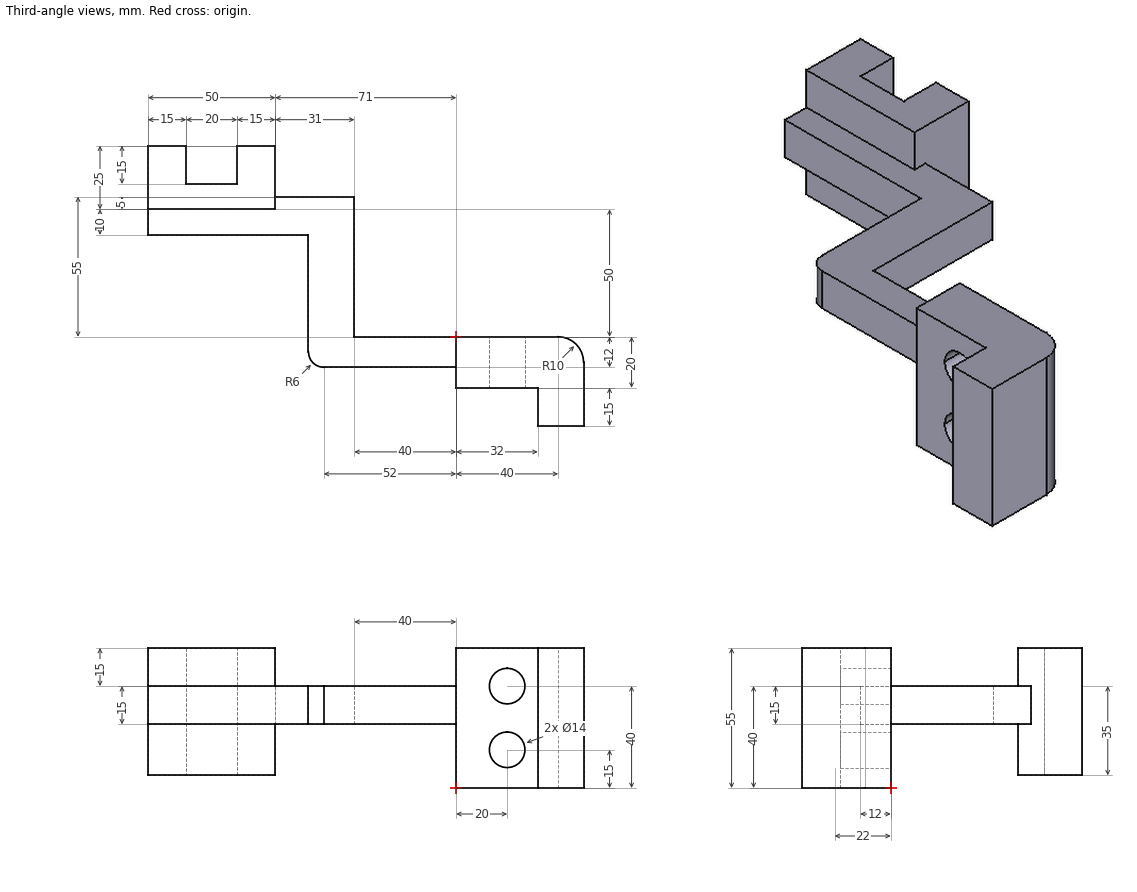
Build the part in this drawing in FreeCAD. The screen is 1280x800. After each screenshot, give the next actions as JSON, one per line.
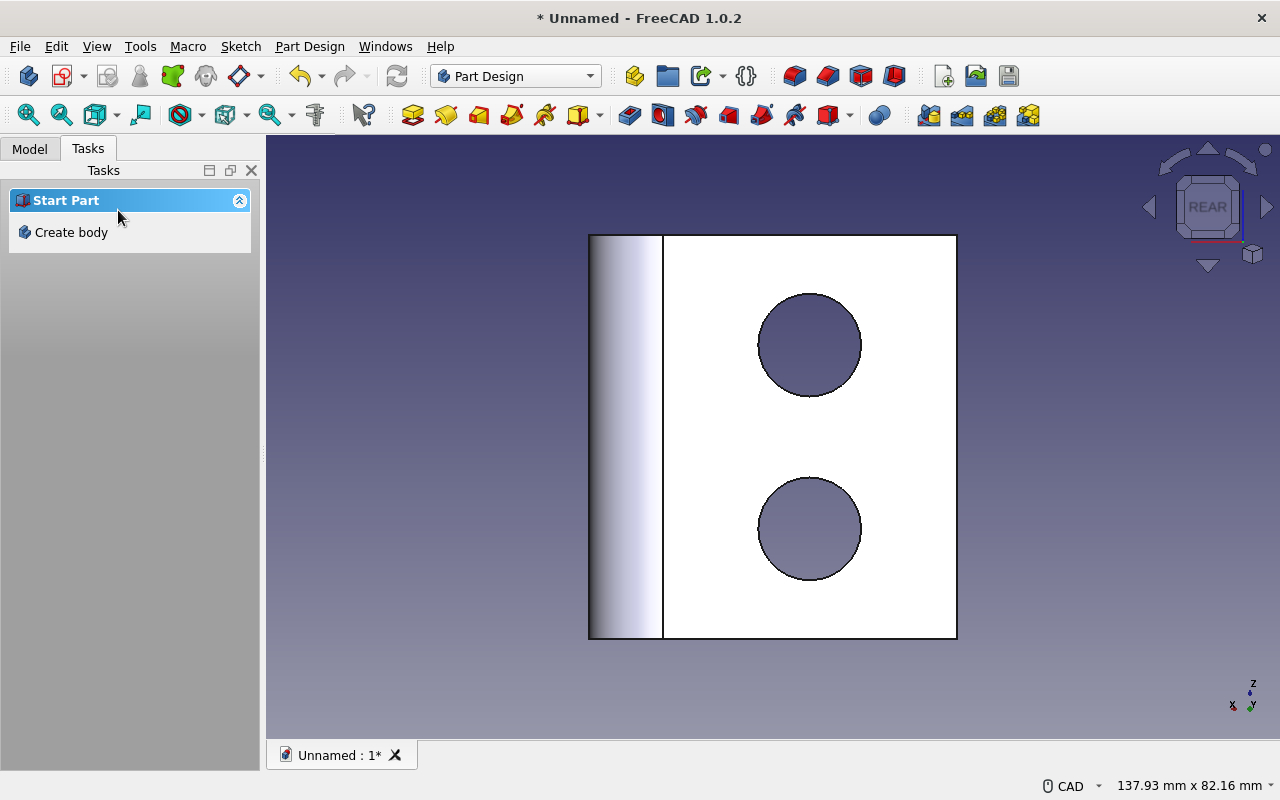
{"action": "left_click", "coordinate": [62, 76]}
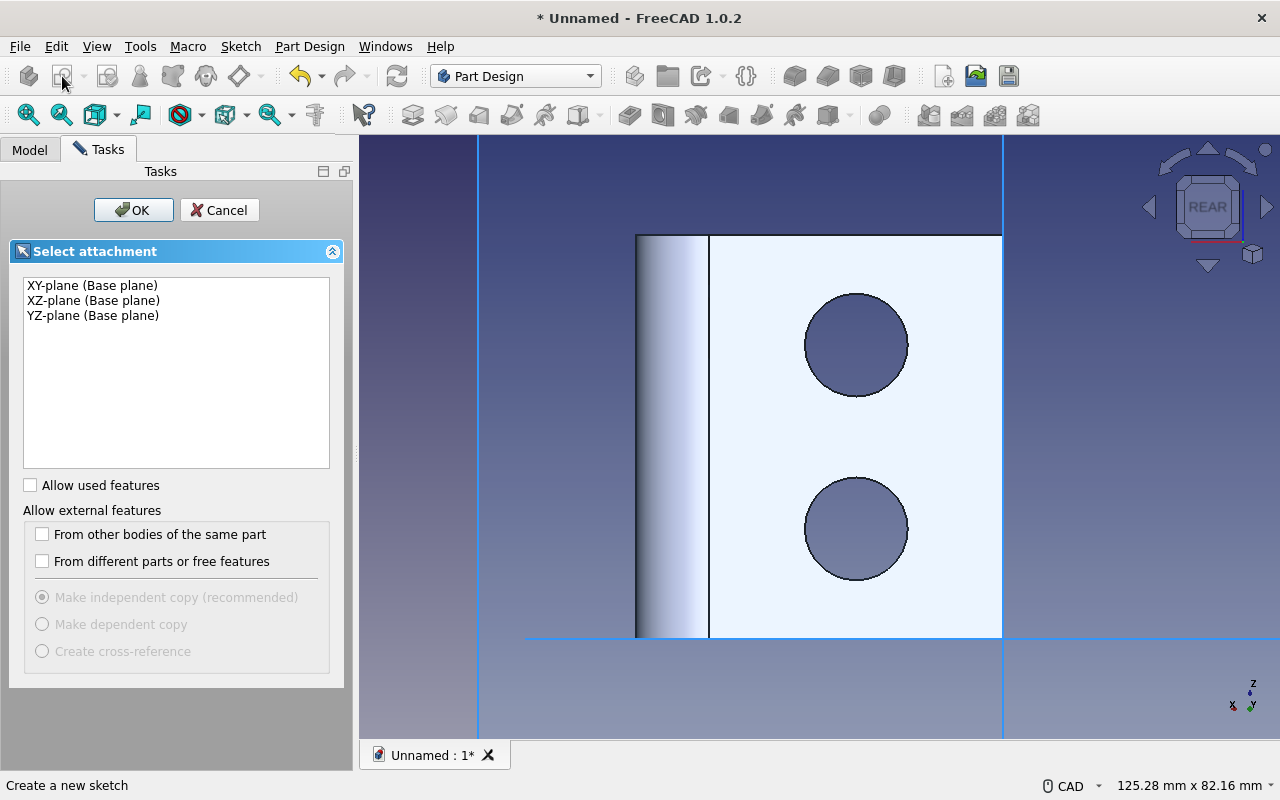
{"action": "left_click", "coordinate": [84, 316]}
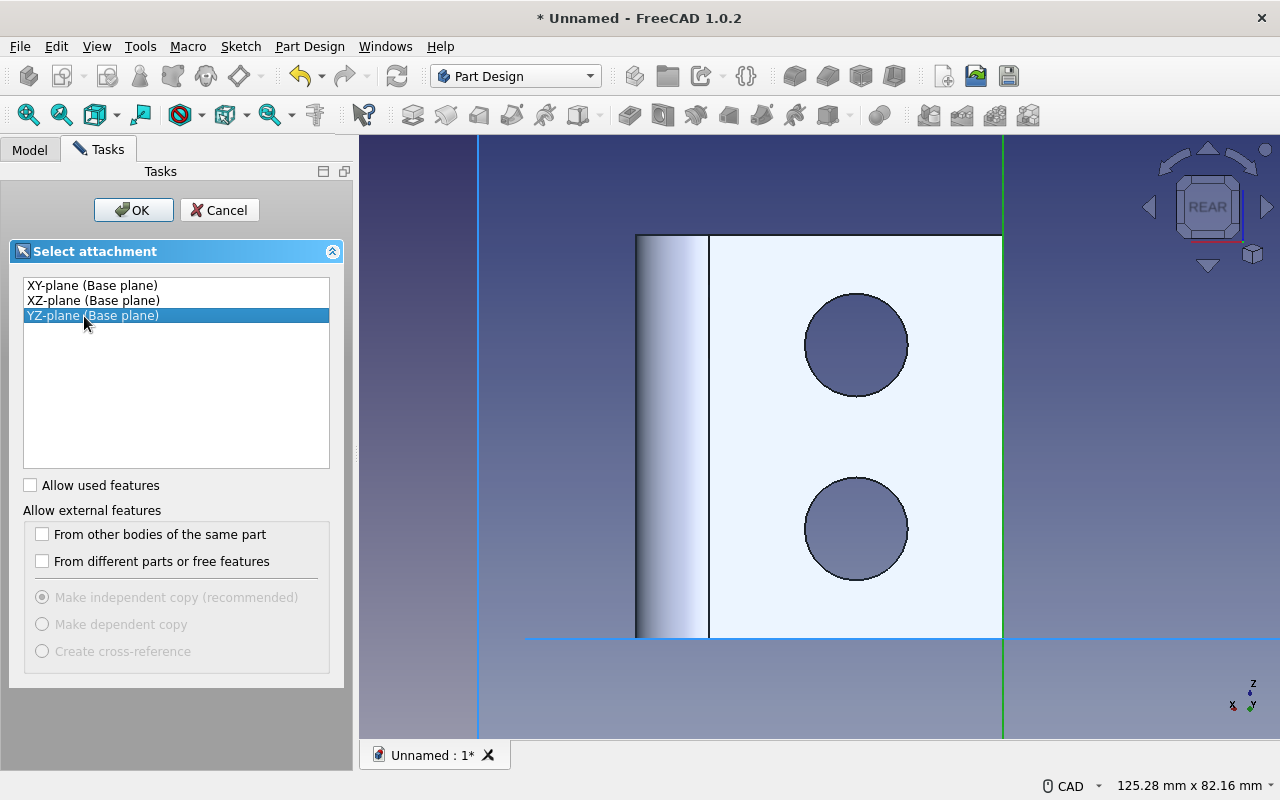
{"action": "left_click", "coordinate": [134, 210]}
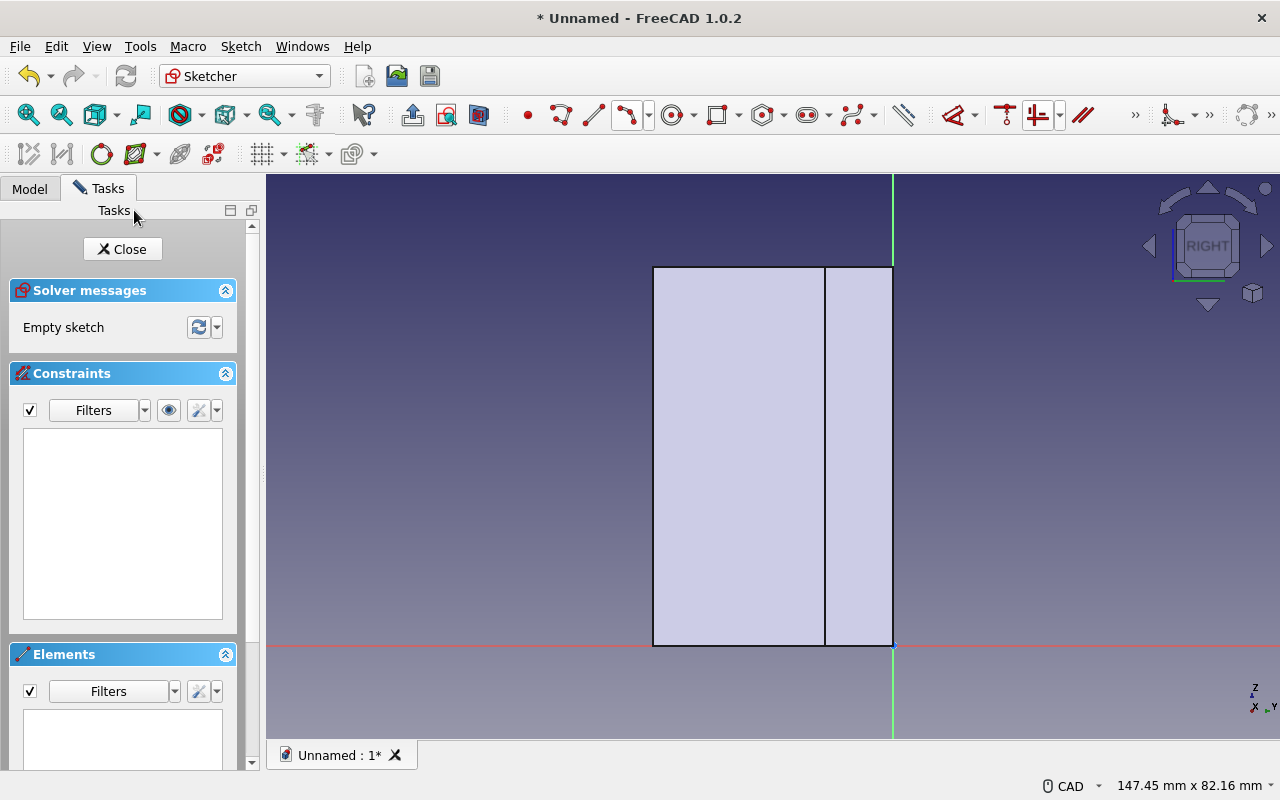
{"action": "left_click", "coordinate": [479, 116]}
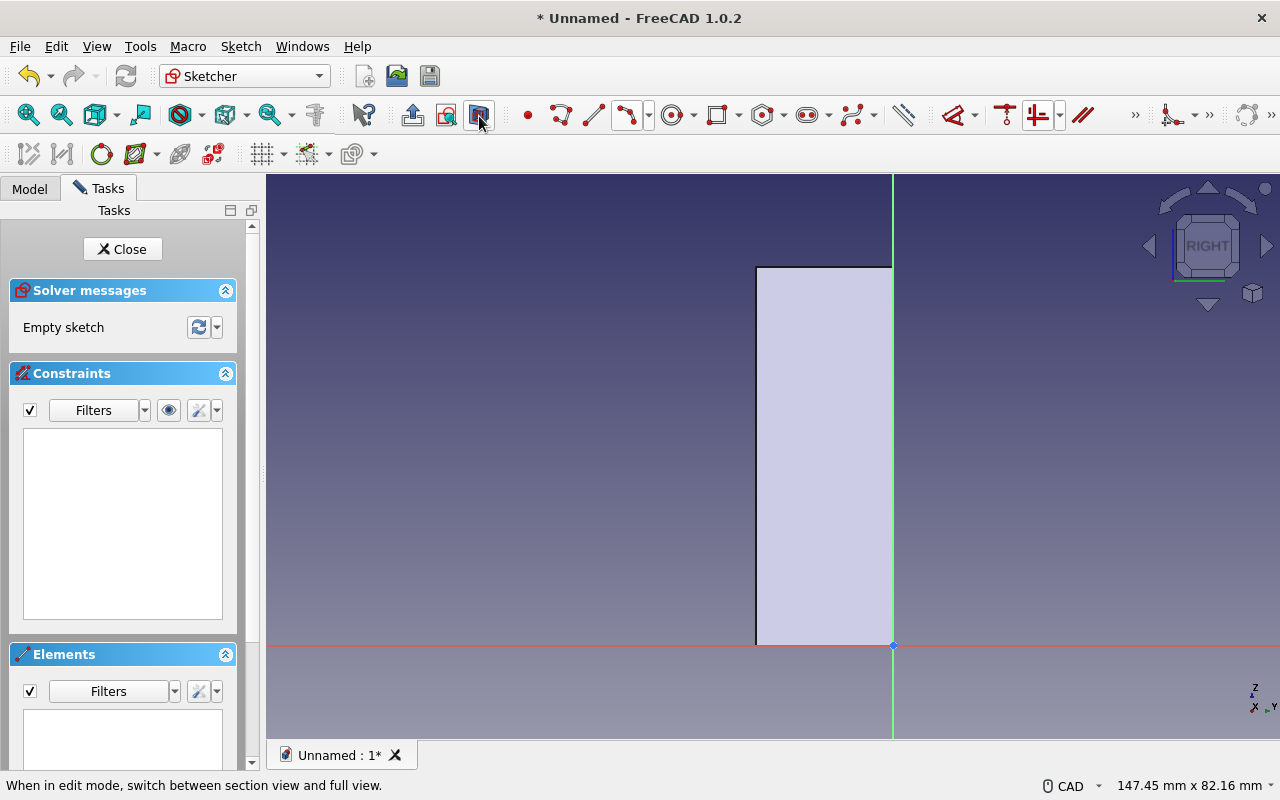
{"action": "scroll", "coordinate": [916, 407], "scroll_direction": "up", "scroll_amount": 6}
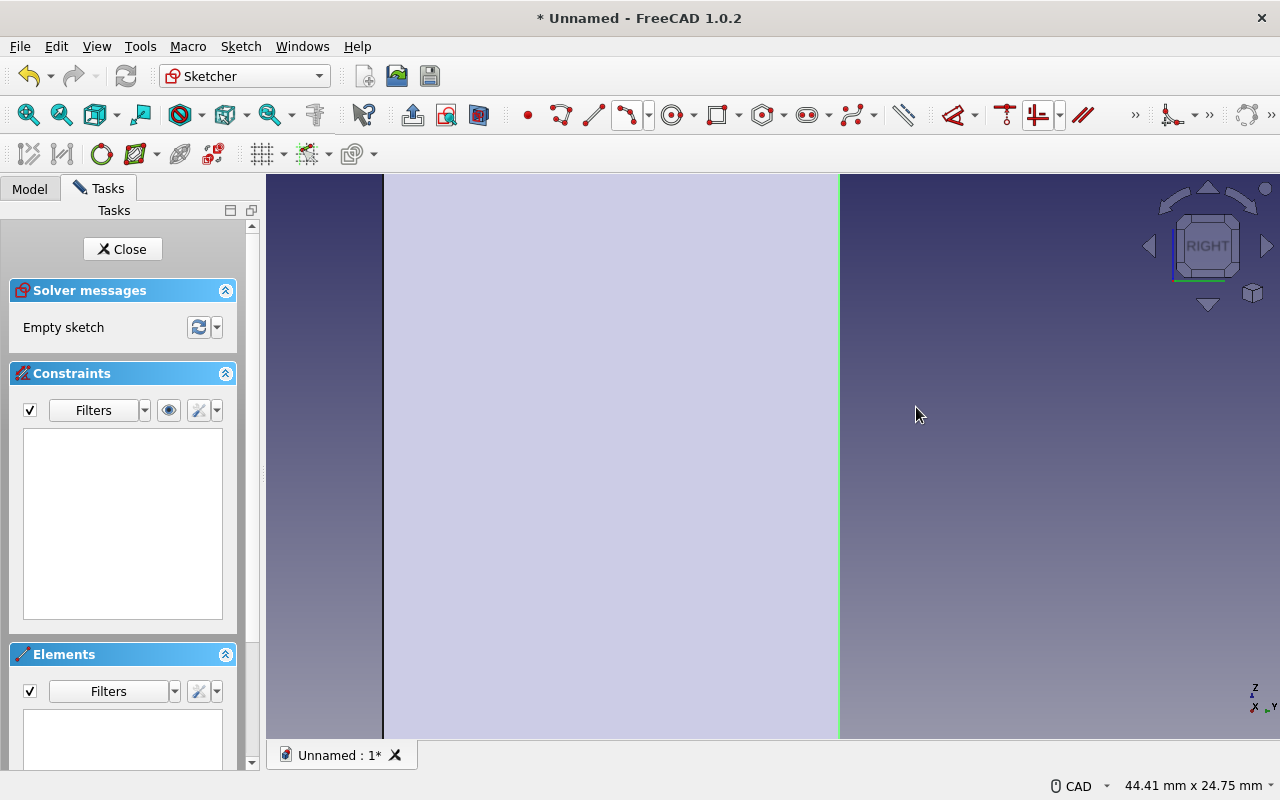
{"action": "left_click", "coordinate": [716, 116]}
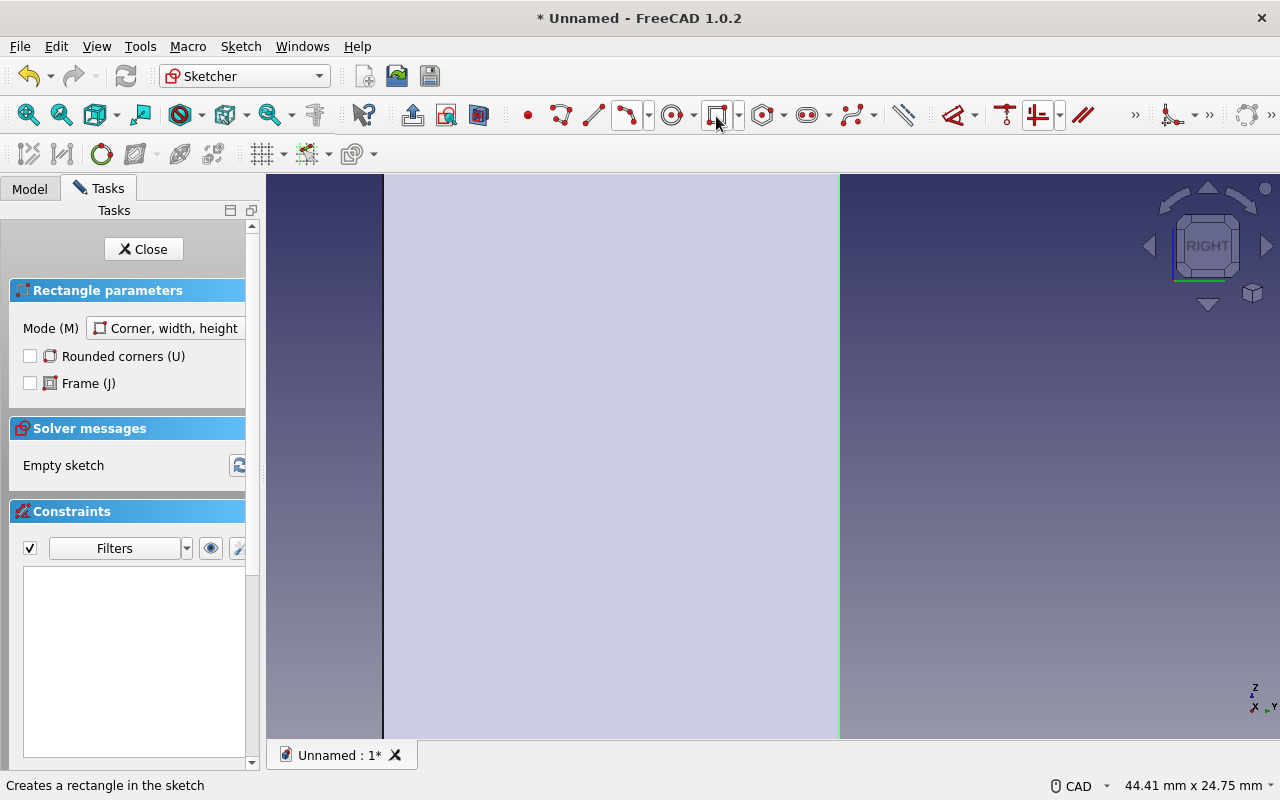
{"action": "left_click", "coordinate": [565, 285]}
{"action": "left_click", "coordinate": [839, 627]}
{"action": "key", "text": "Escape"}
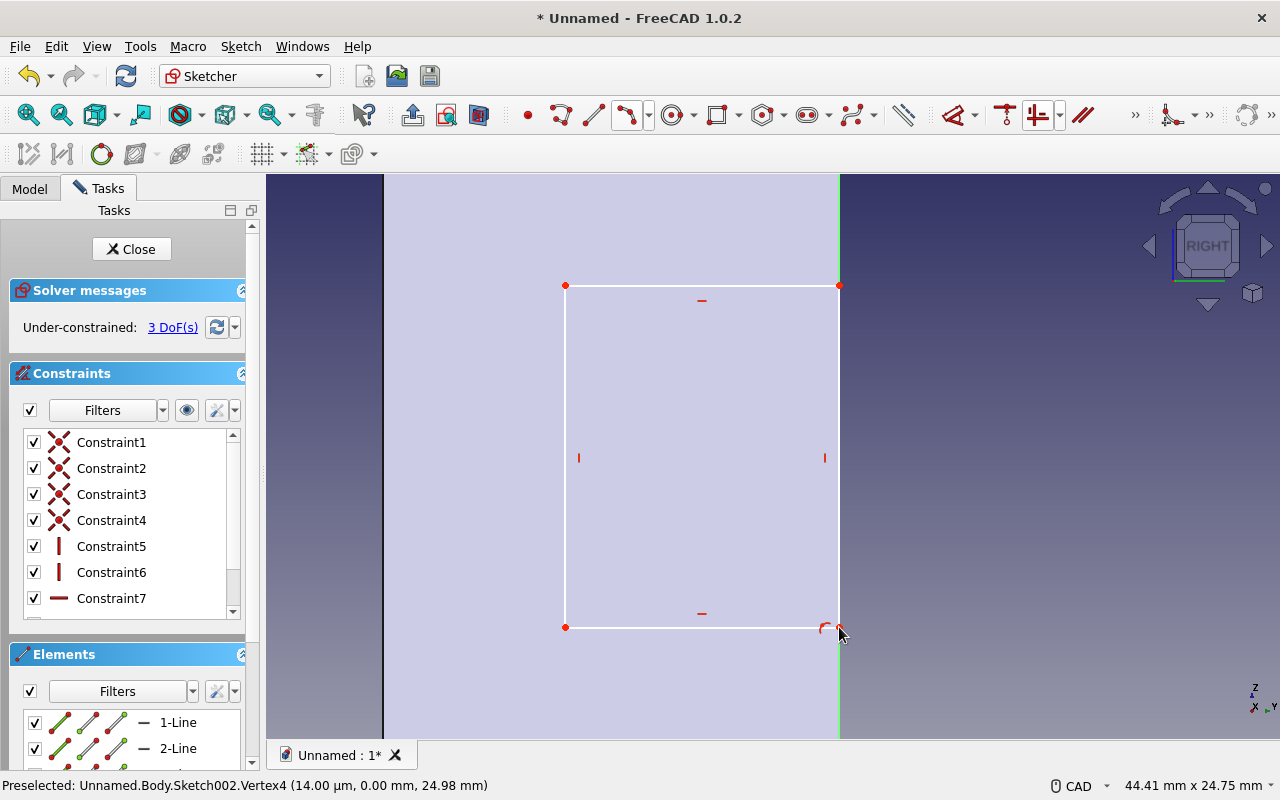
{"action": "left_click", "coordinate": [952, 116]}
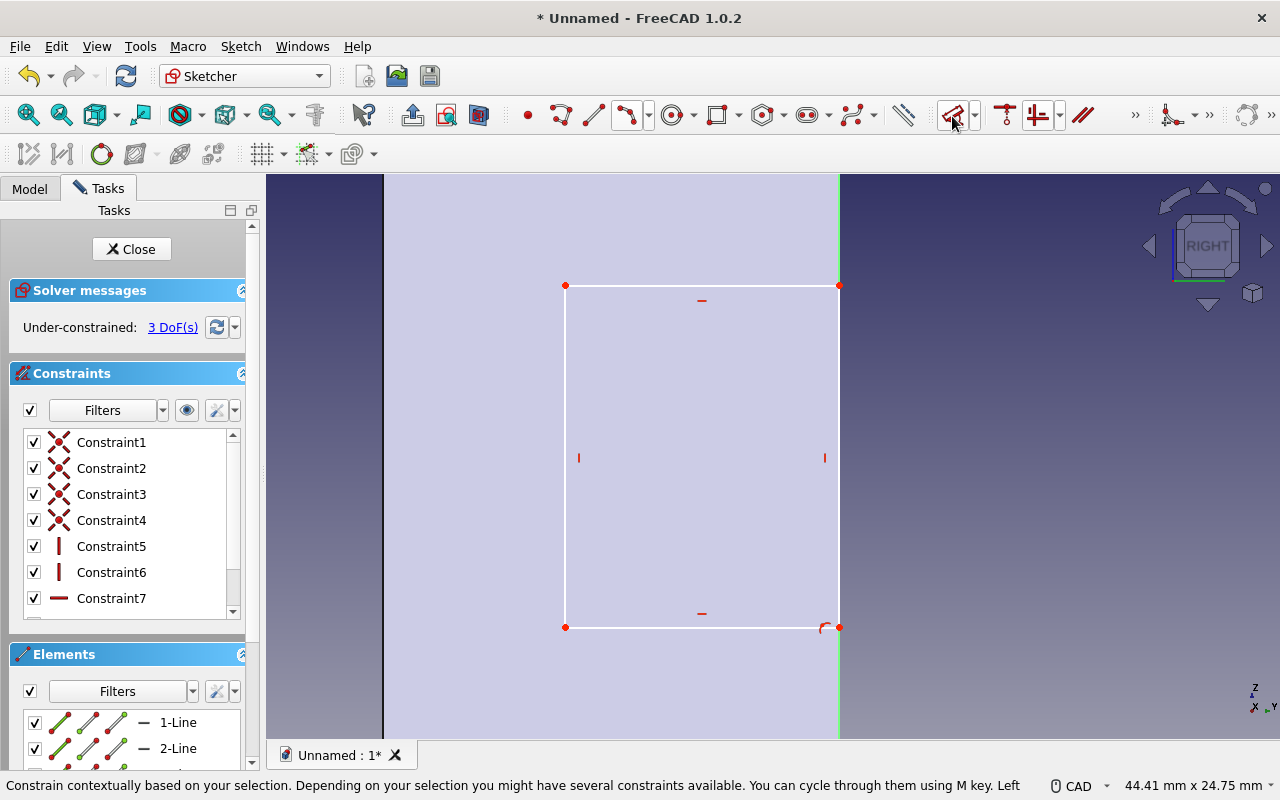
{"action": "left_click", "coordinate": [565, 389]}
{"action": "left_click", "coordinate": [531, 457]}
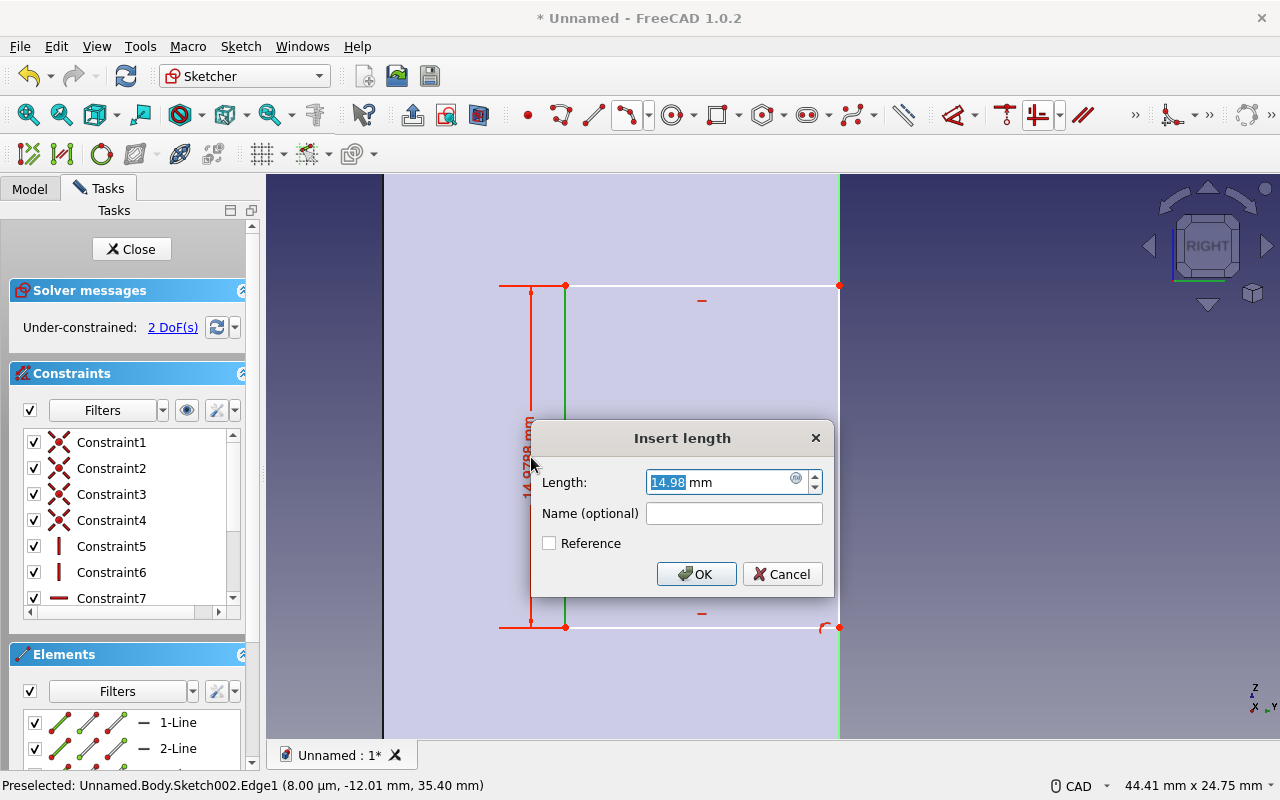
{"action": "type", "text": "15"}
{"action": "key", "text": "Return"}